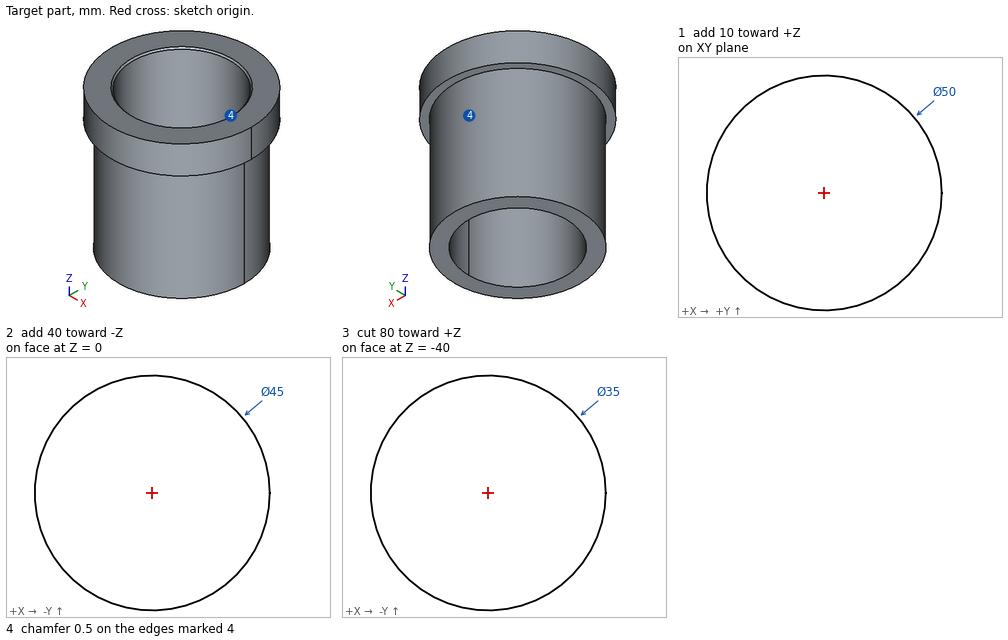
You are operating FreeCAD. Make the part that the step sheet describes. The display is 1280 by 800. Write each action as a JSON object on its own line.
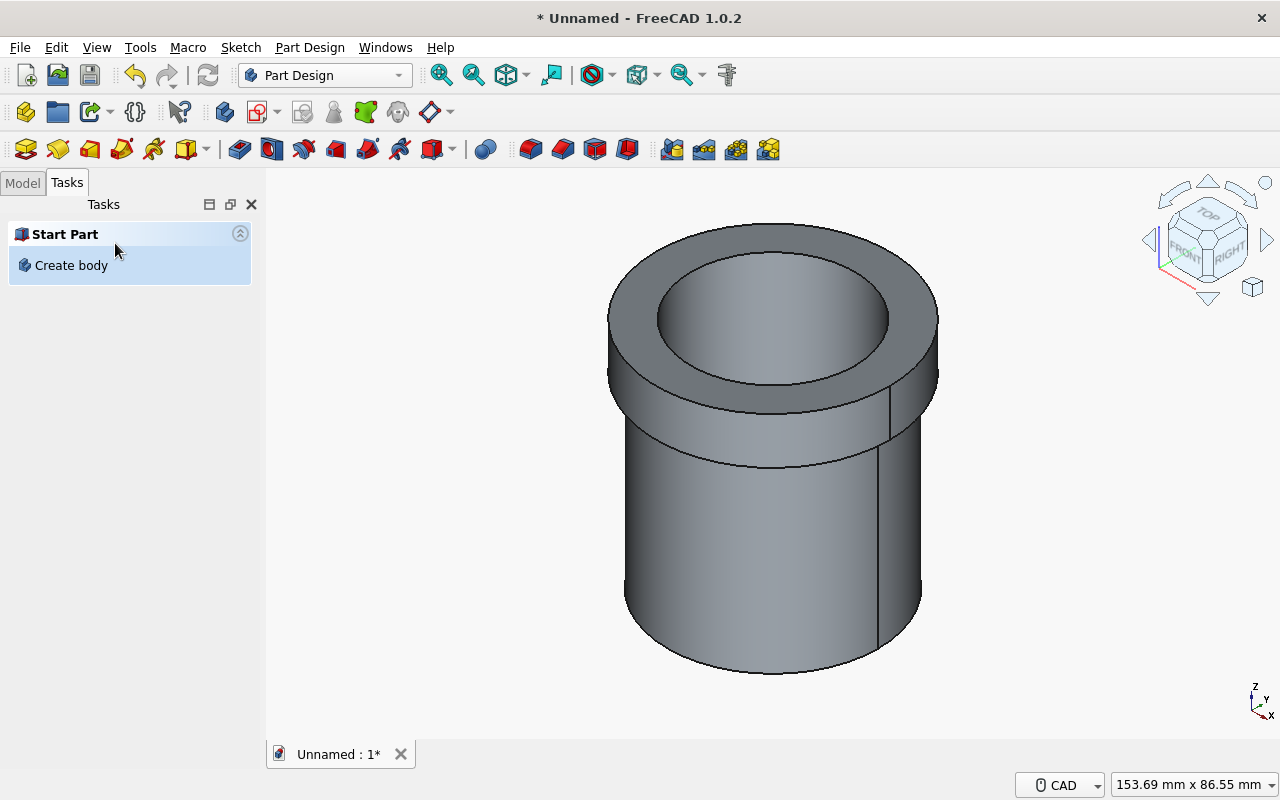
{"action": "left_click", "coordinate": [691, 271]}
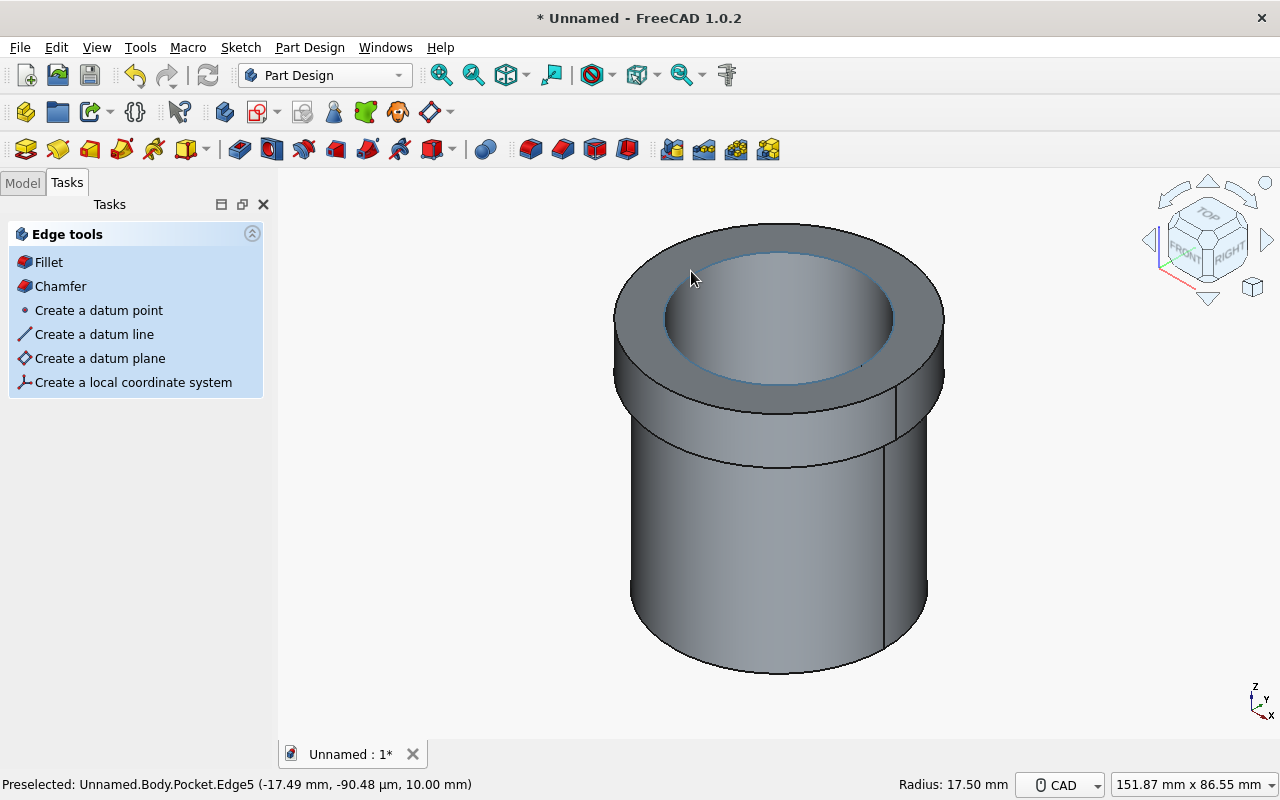
{"action": "left_click", "coordinate": [564, 150]}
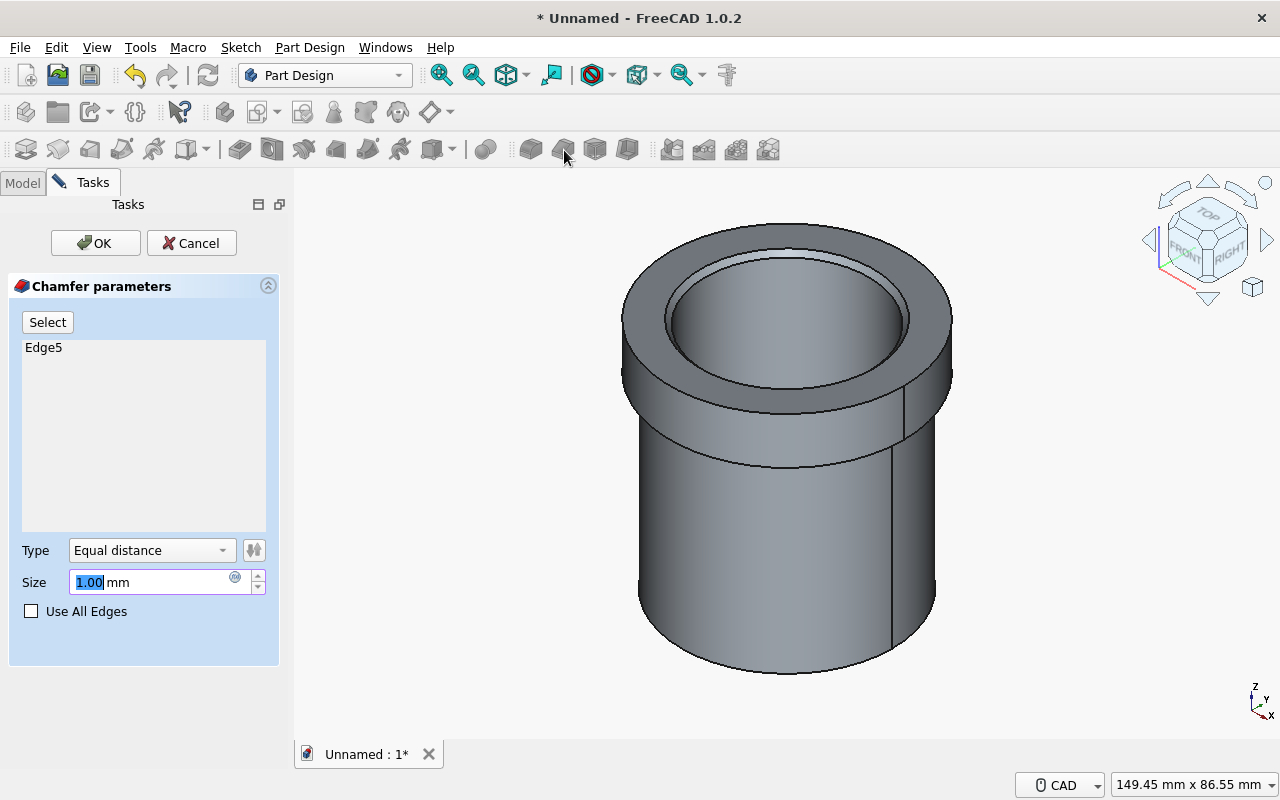
{"action": "type", "text": "0.5"}
{"action": "key", "text": "Tab"}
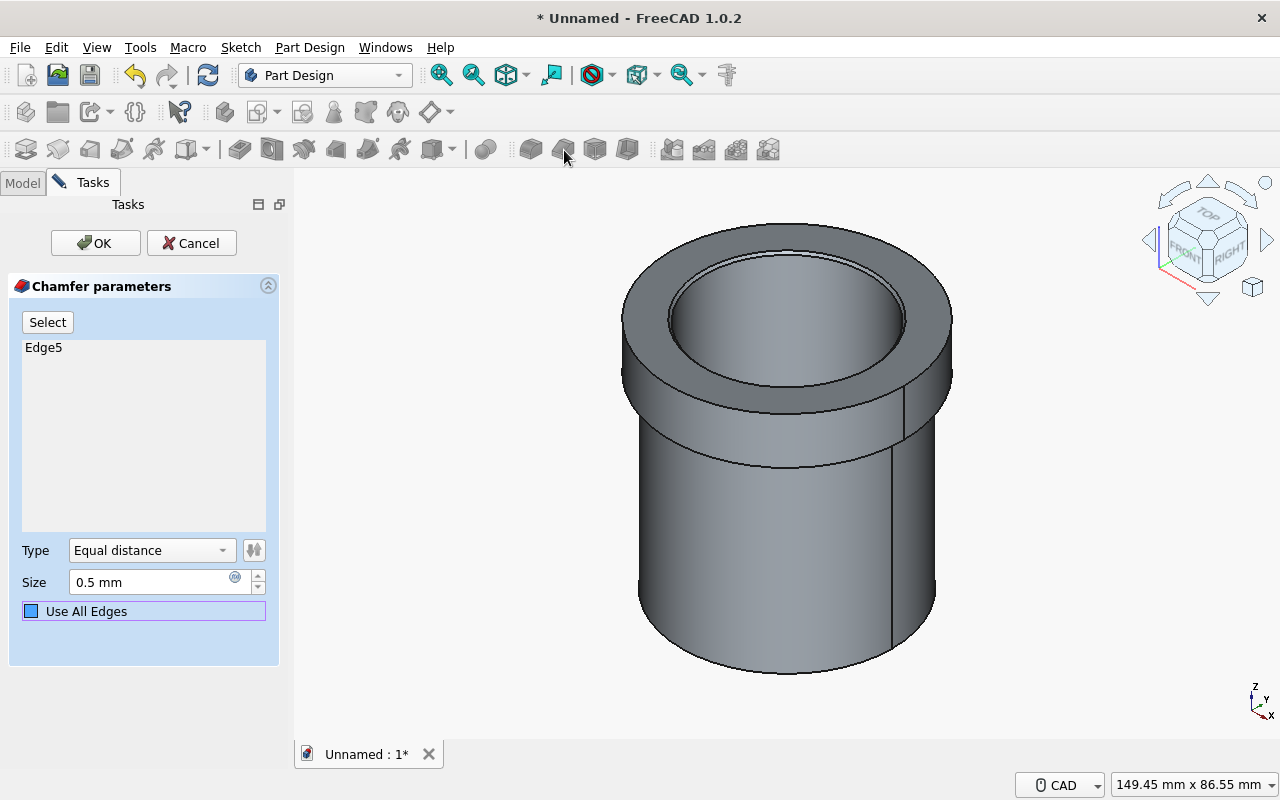
{"action": "left_click", "coordinate": [96, 243]}